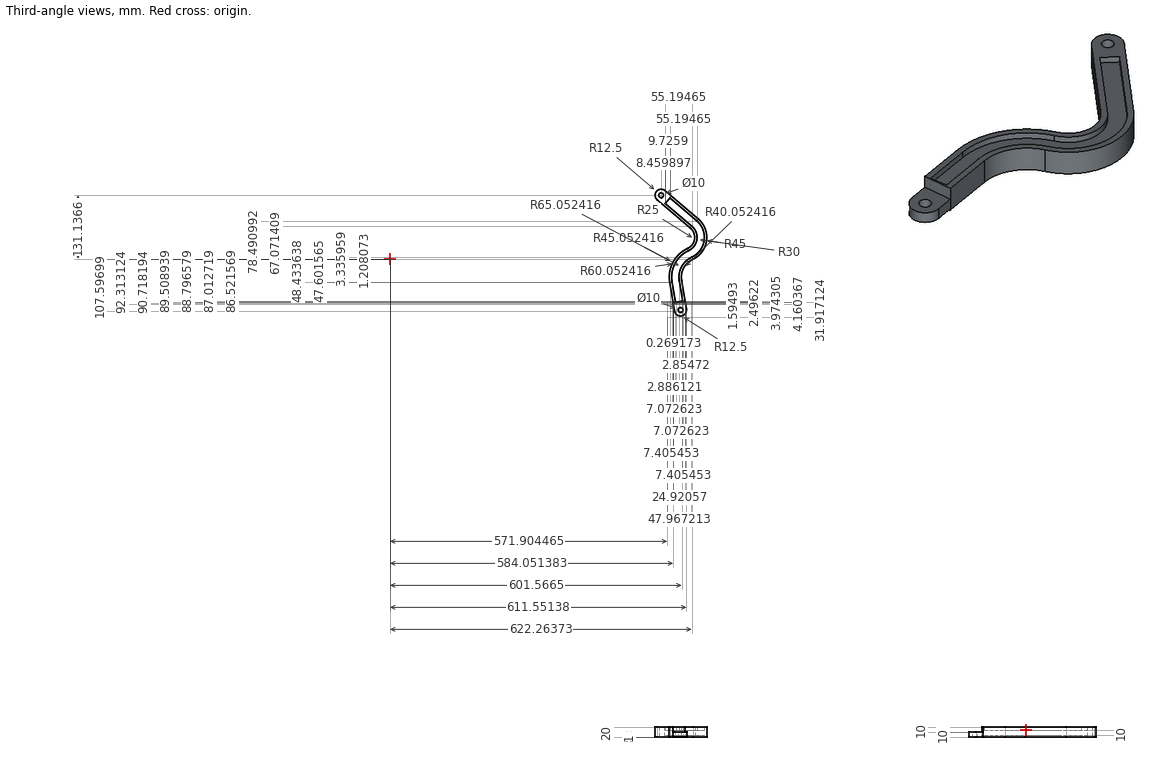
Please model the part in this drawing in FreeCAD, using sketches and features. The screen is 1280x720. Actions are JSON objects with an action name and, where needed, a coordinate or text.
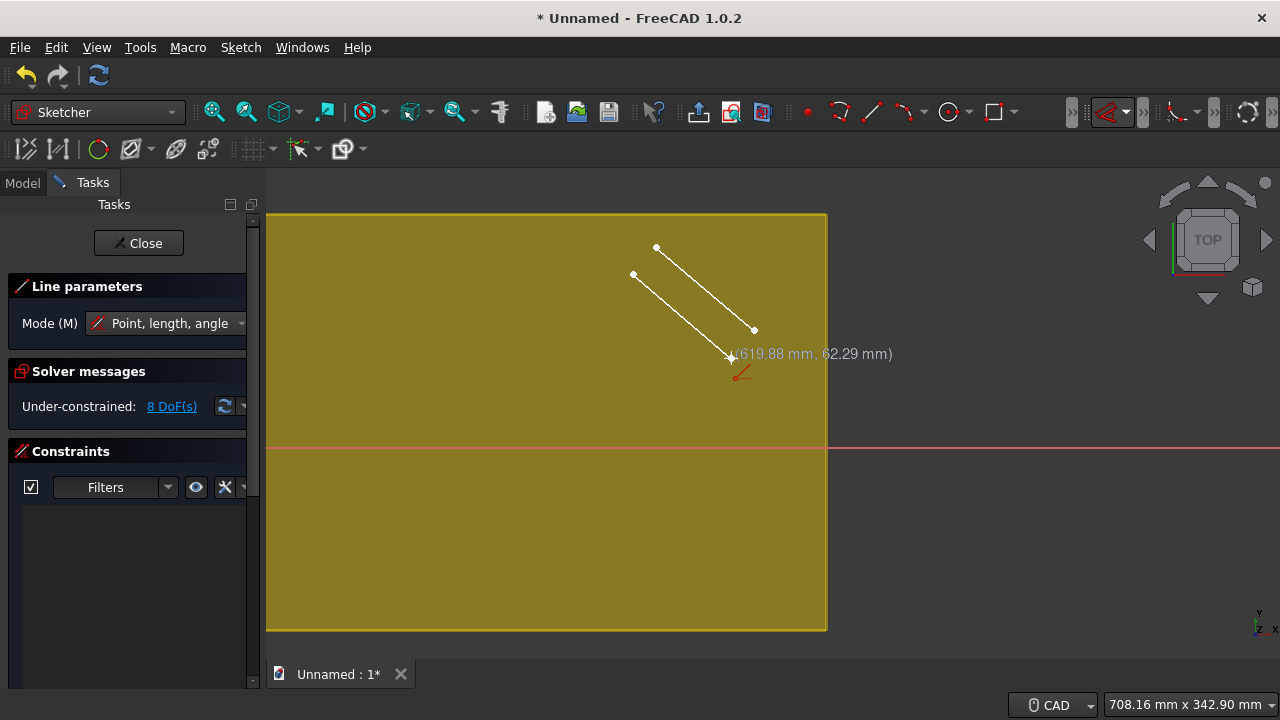
{"action": "left_click", "coordinate": [840, 112]}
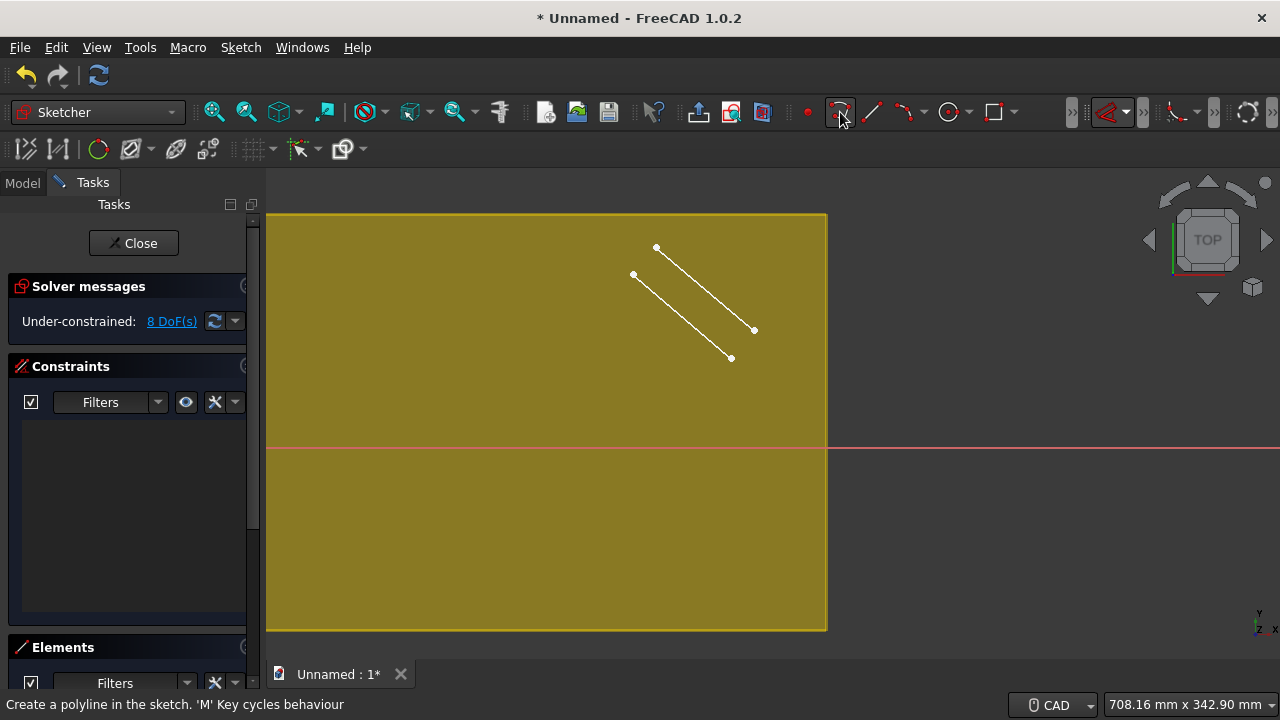
{"action": "left_click", "coordinate": [669, 518]}
{"action": "left_click", "coordinate": [680, 580]}
{"action": "left_click", "coordinate": [715, 574]}
{"action": "left_click", "coordinate": [705, 512]}
{"action": "right_click", "coordinate": [705, 512]}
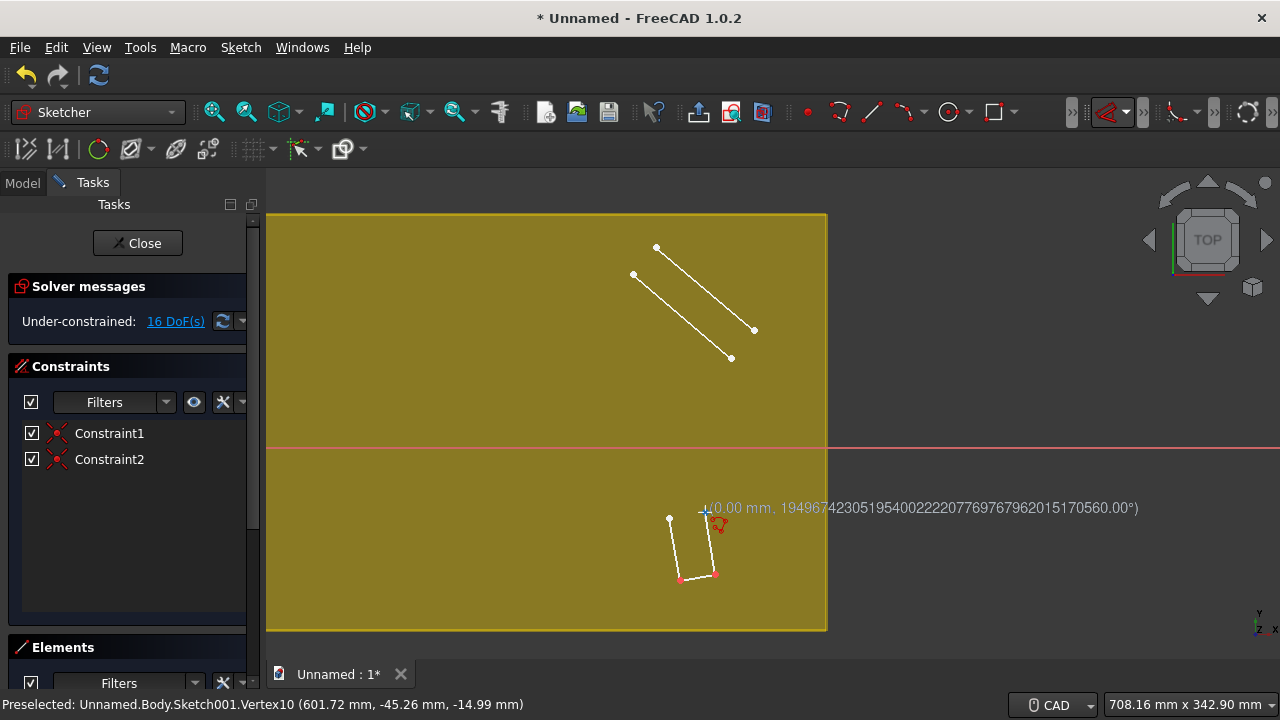
{"action": "left_click", "coordinate": [904, 112]}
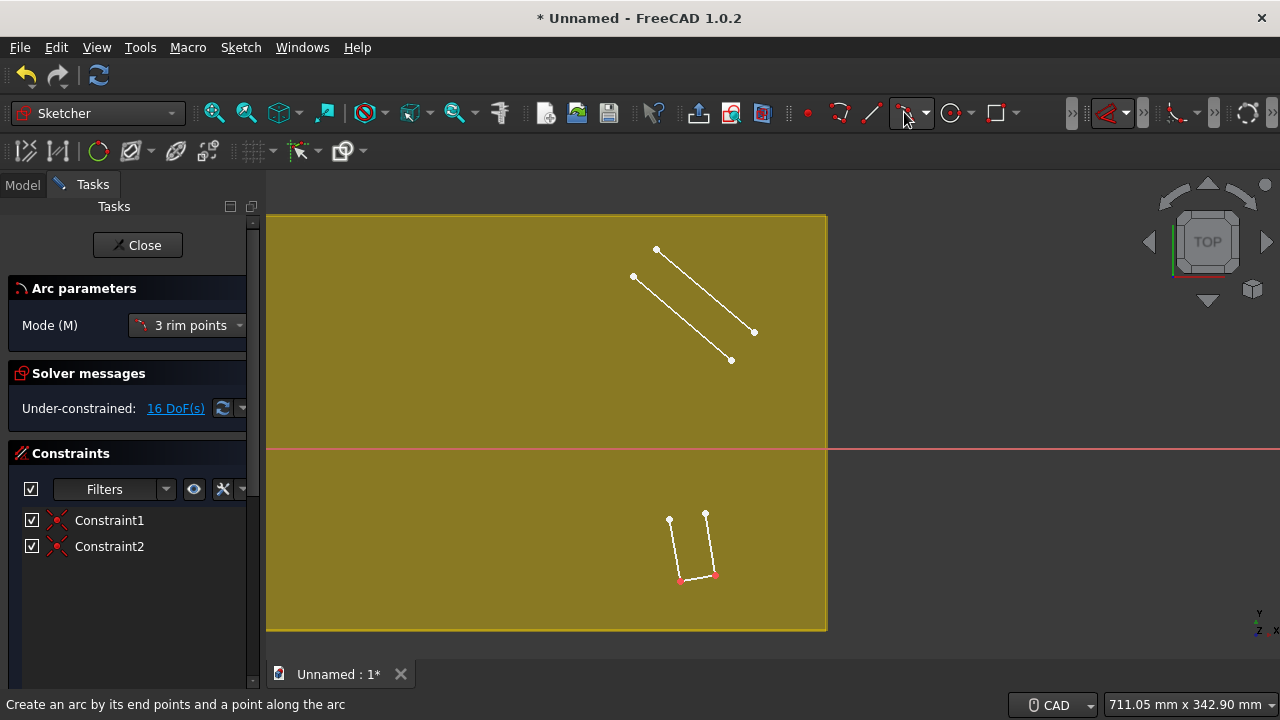
{"action": "left_click", "coordinate": [656, 250]}
{"action": "left_click", "coordinate": [634, 277]}
{"action": "left_click", "coordinate": [631, 250]}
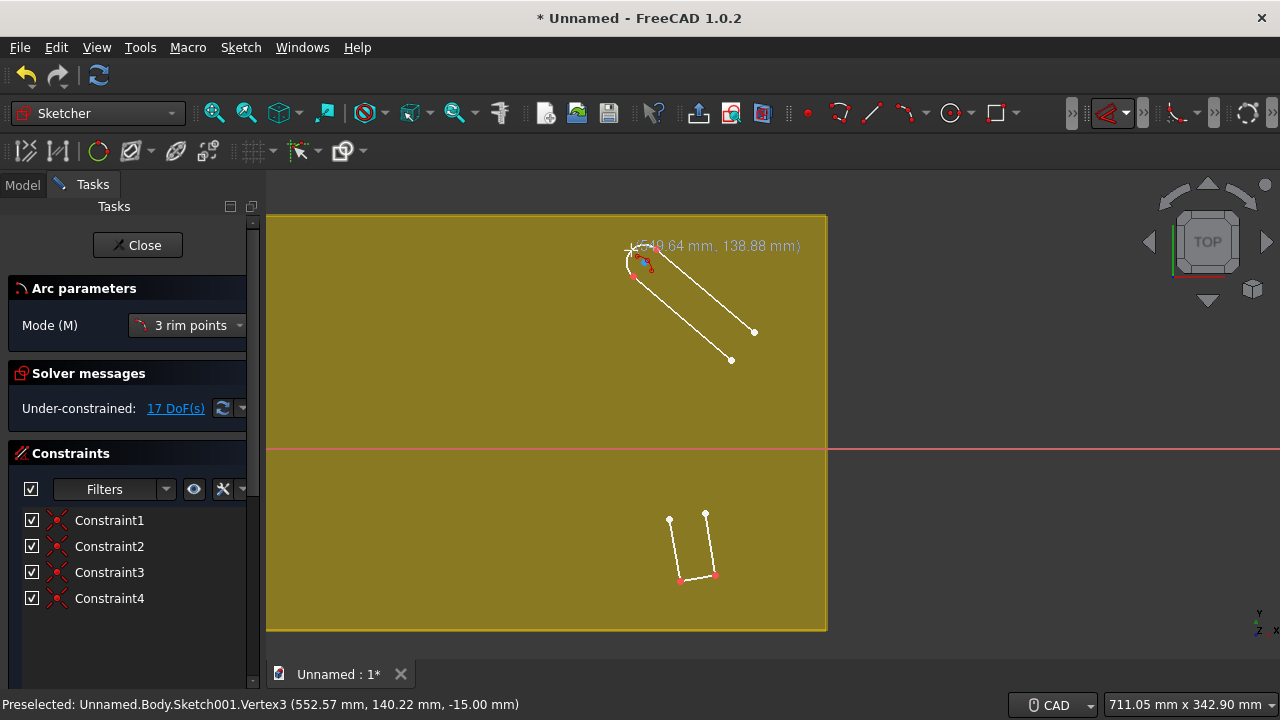
{"action": "left_click", "coordinate": [731, 360]}
{"action": "left_click", "coordinate": [723, 418]}
{"action": "left_click", "coordinate": [743, 391]}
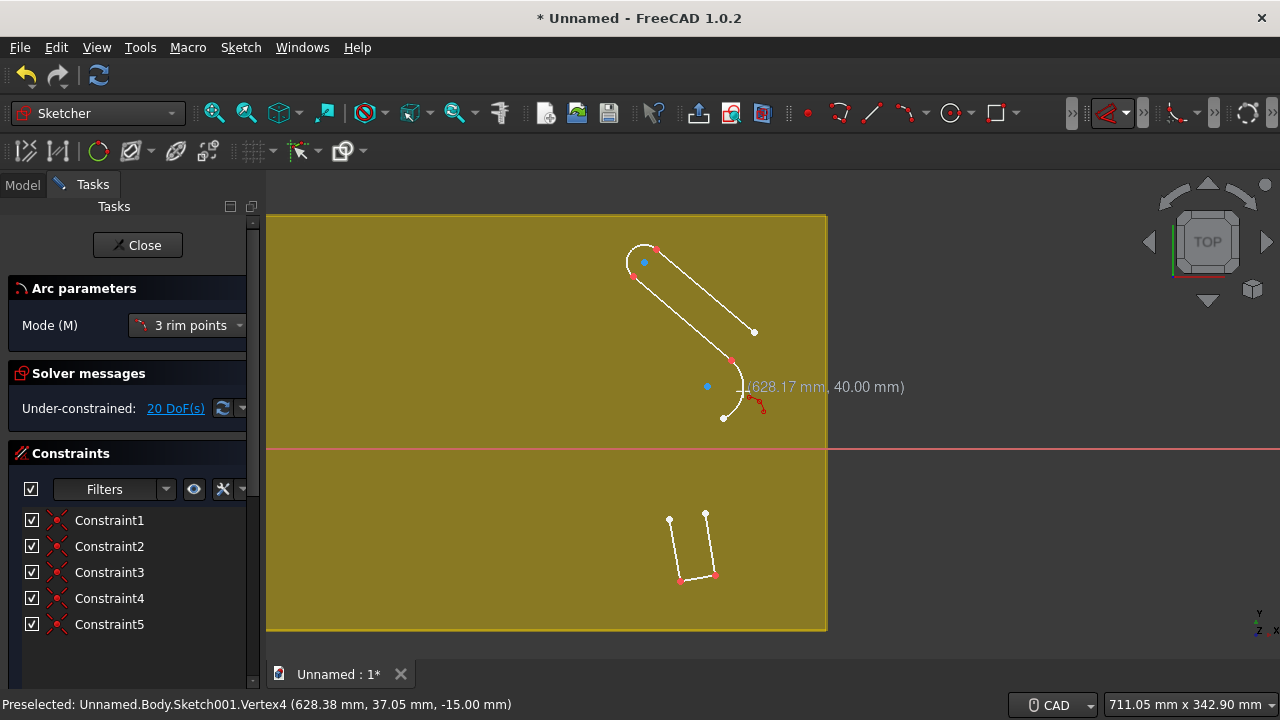
{"action": "left_click", "coordinate": [723, 419]}
{"action": "left_click", "coordinate": [669, 520]}
{"action": "left_click", "coordinate": [674, 470]}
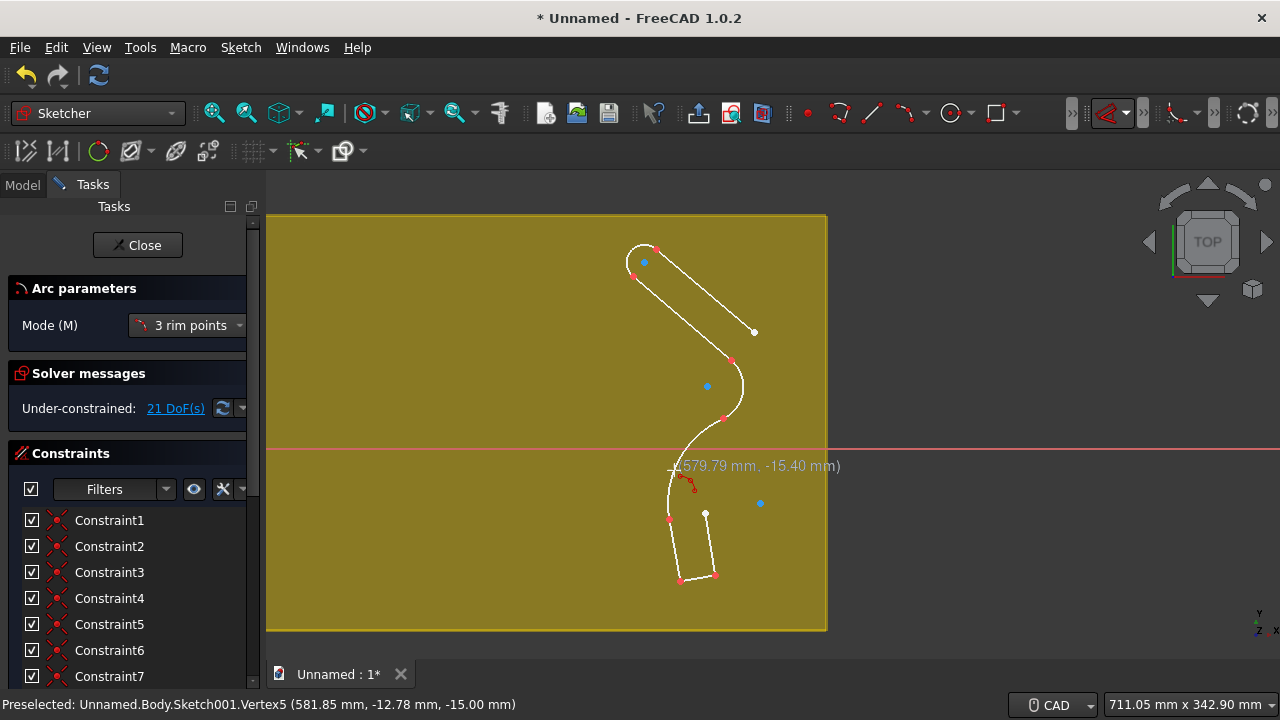
{"action": "left_click", "coordinate": [705, 514]}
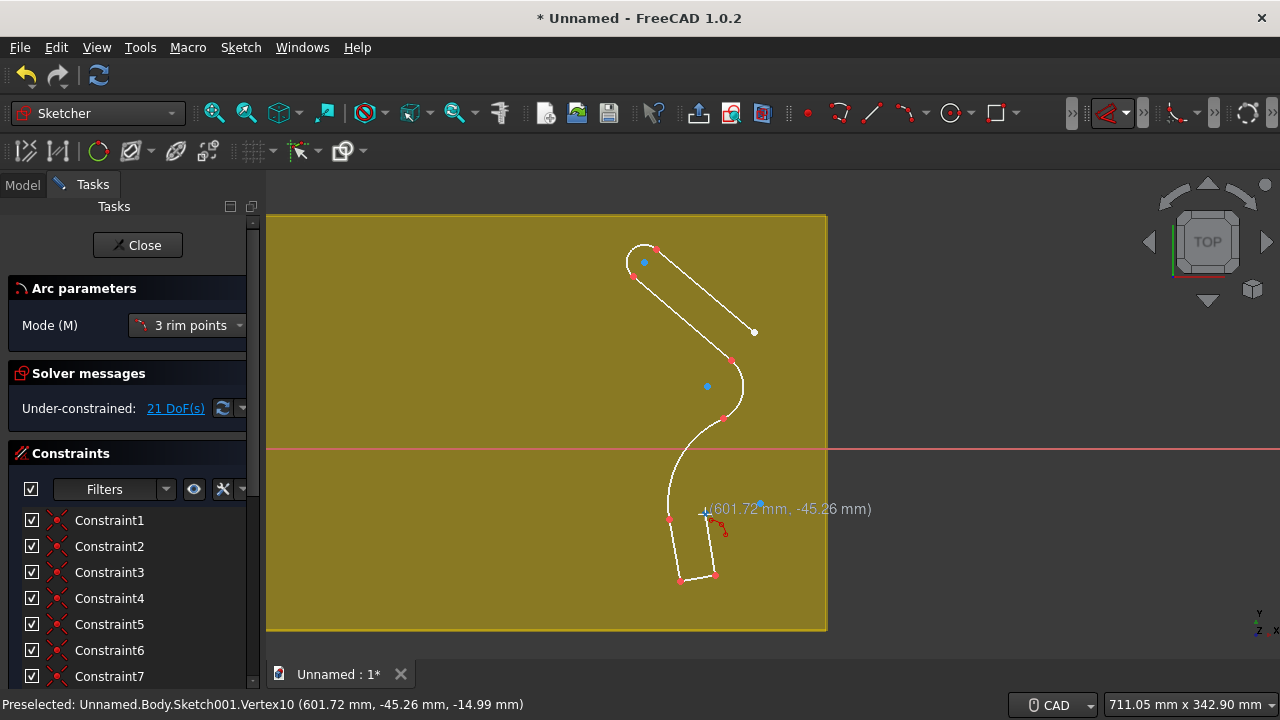
{"action": "scroll", "coordinate": [738, 451], "scroll_direction": "up", "scroll_amount": 12}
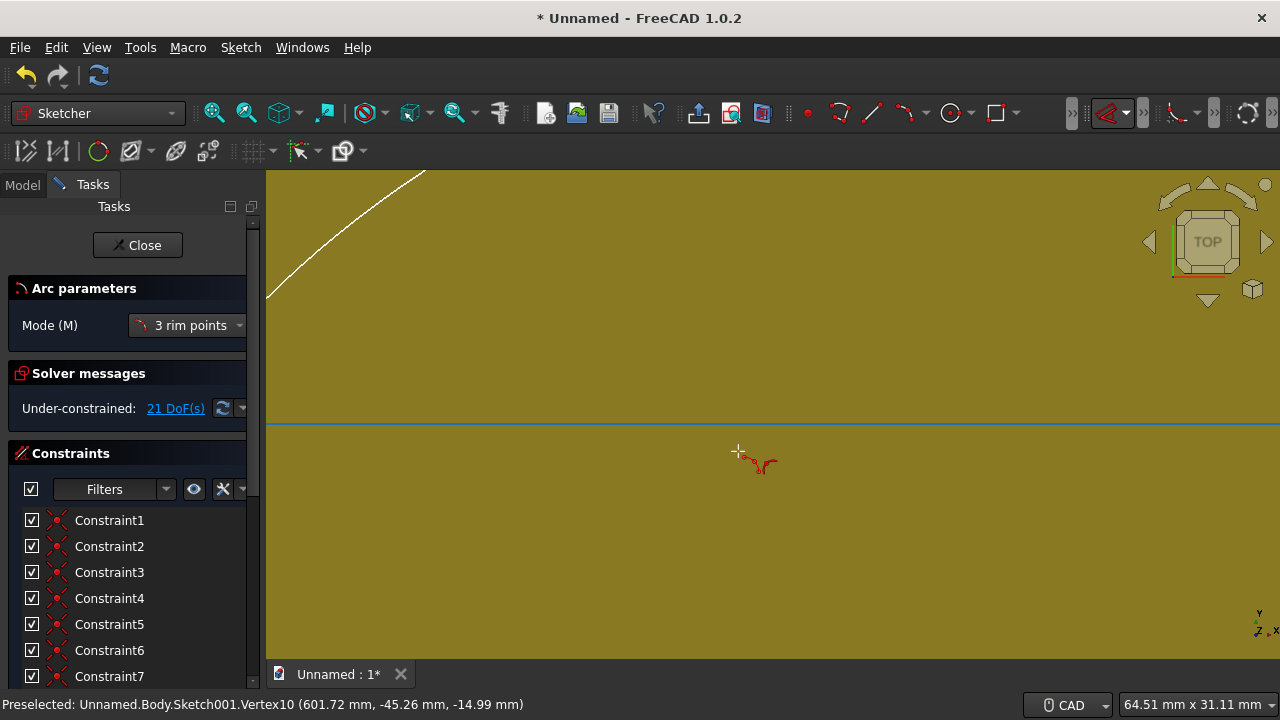
{"action": "left_click", "coordinate": [728, 443]}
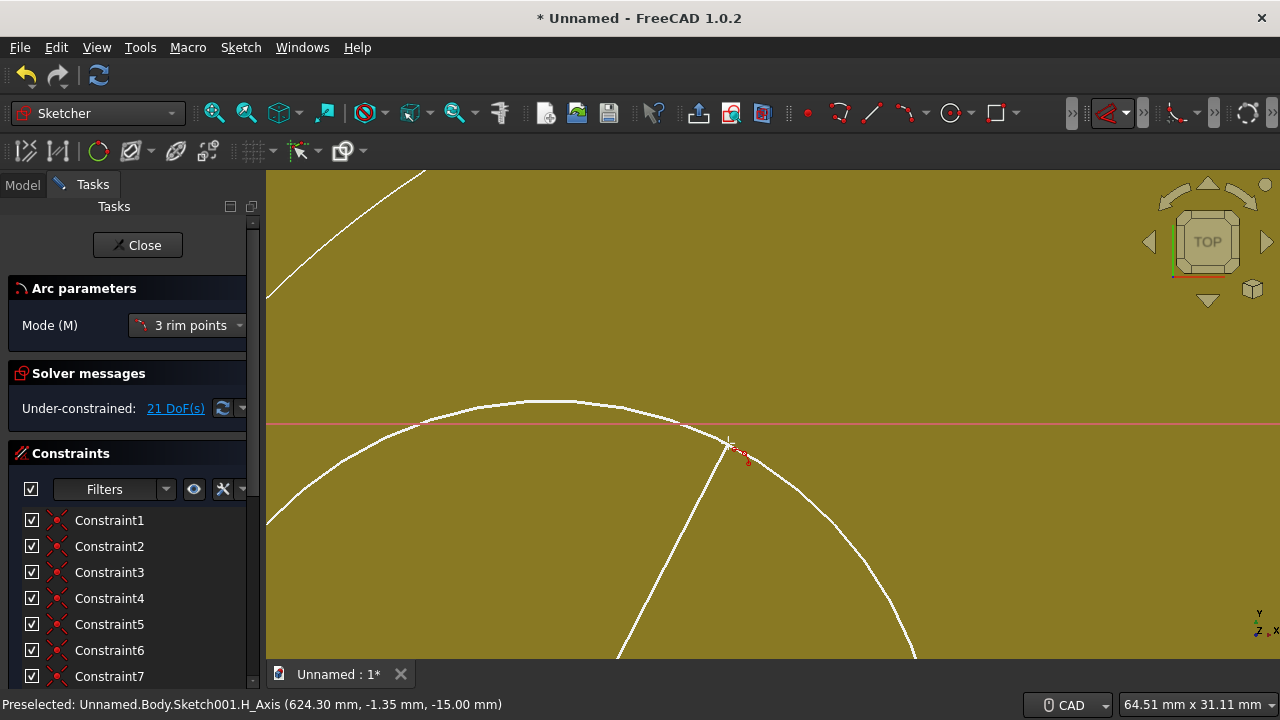
{"action": "scroll", "coordinate": [738, 451], "scroll_direction": "down", "scroll_amount": 12}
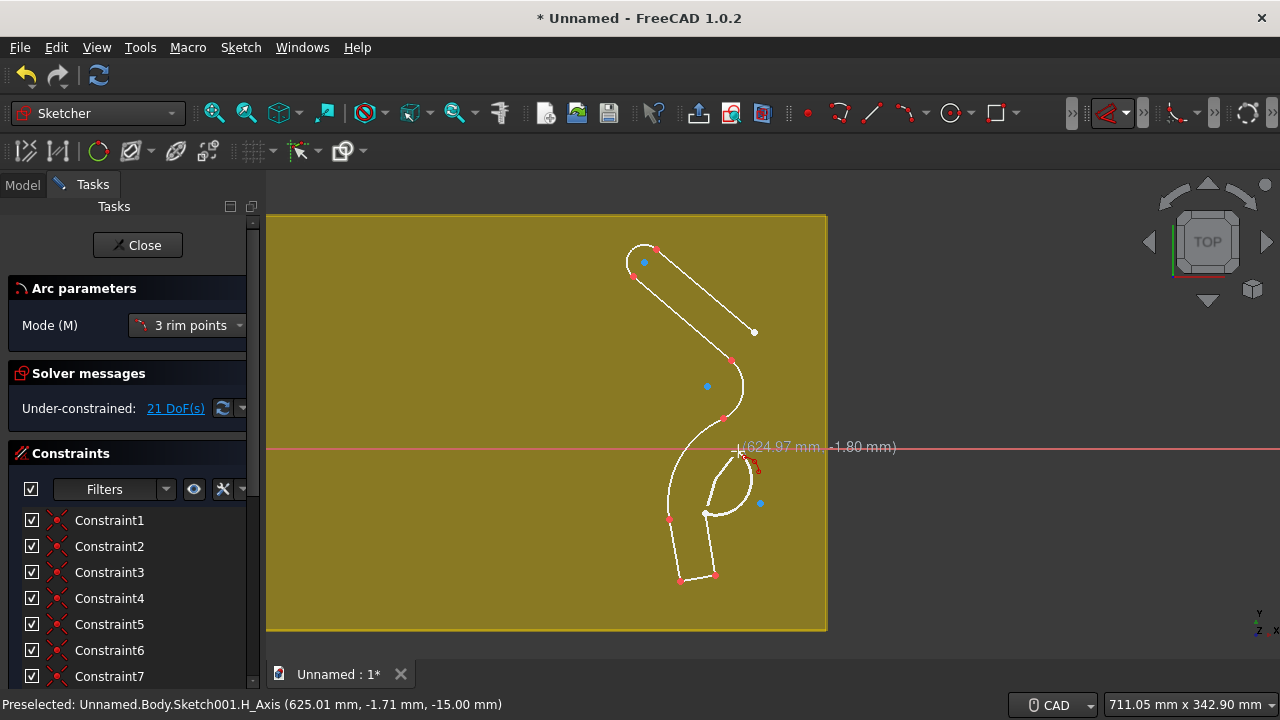
{"action": "scroll", "coordinate": [711, 476], "scroll_direction": "up", "scroll_amount": 2}